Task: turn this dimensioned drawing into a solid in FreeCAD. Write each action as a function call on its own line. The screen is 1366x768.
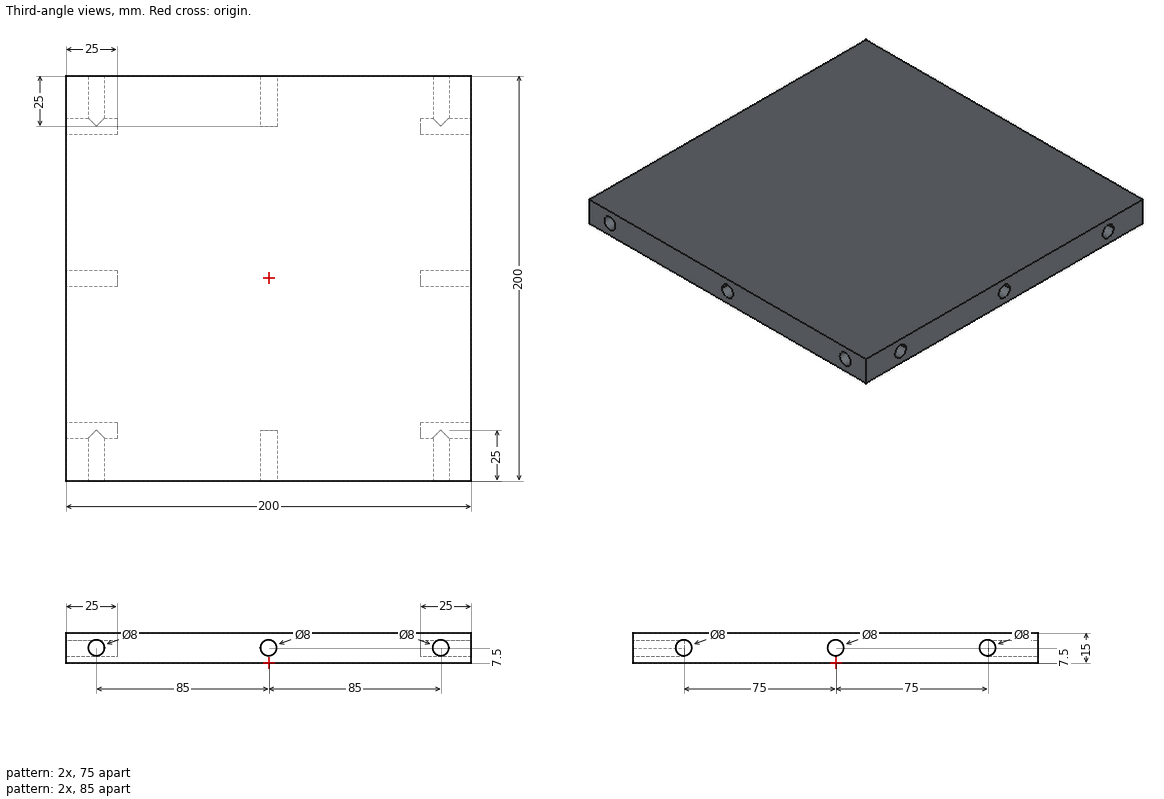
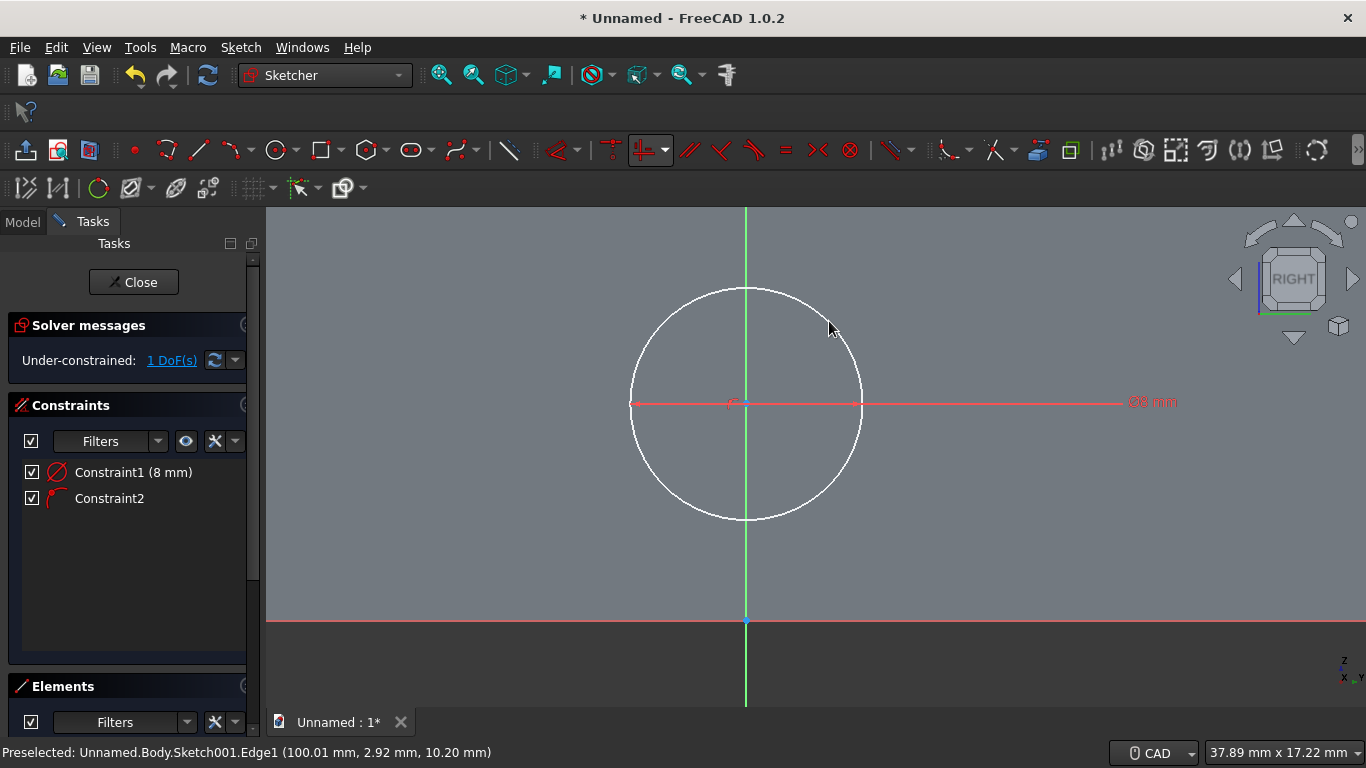
click(556, 150)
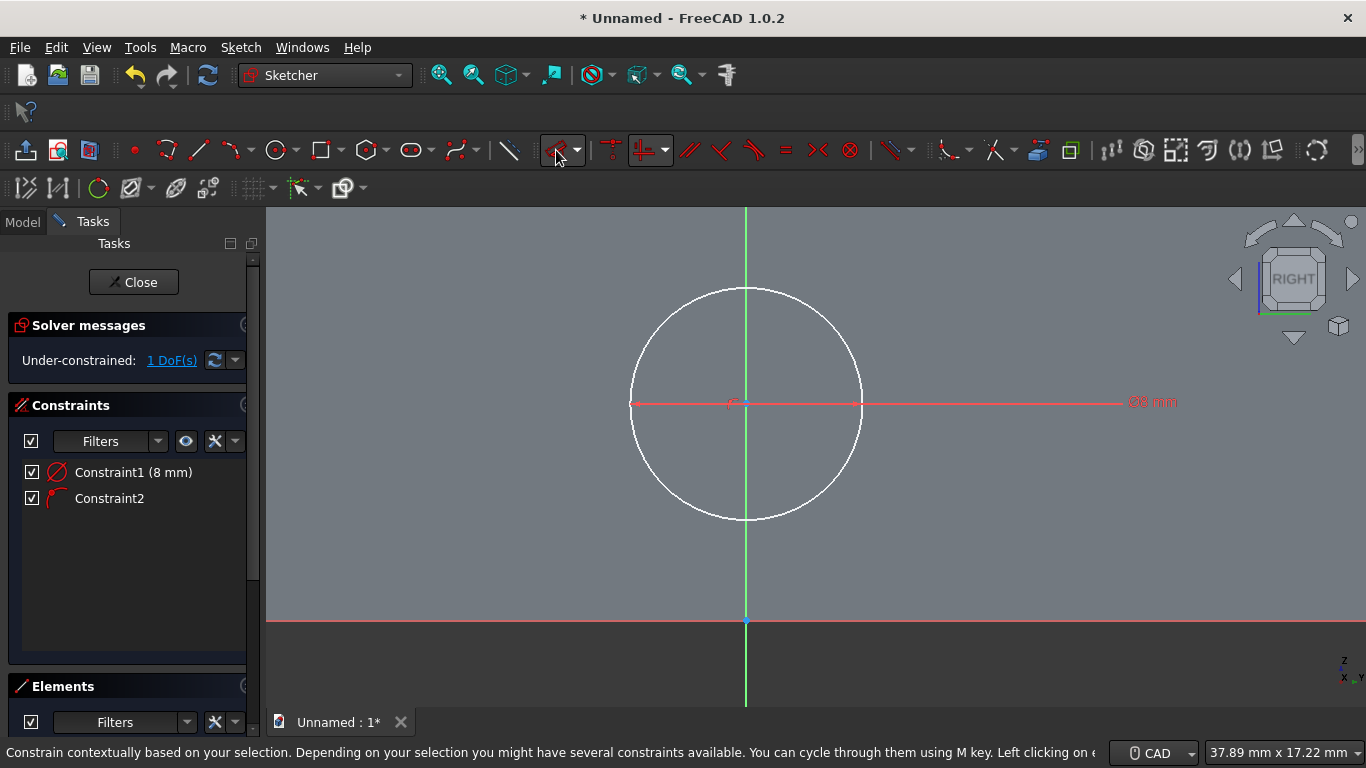
click(746, 404)
click(780, 462)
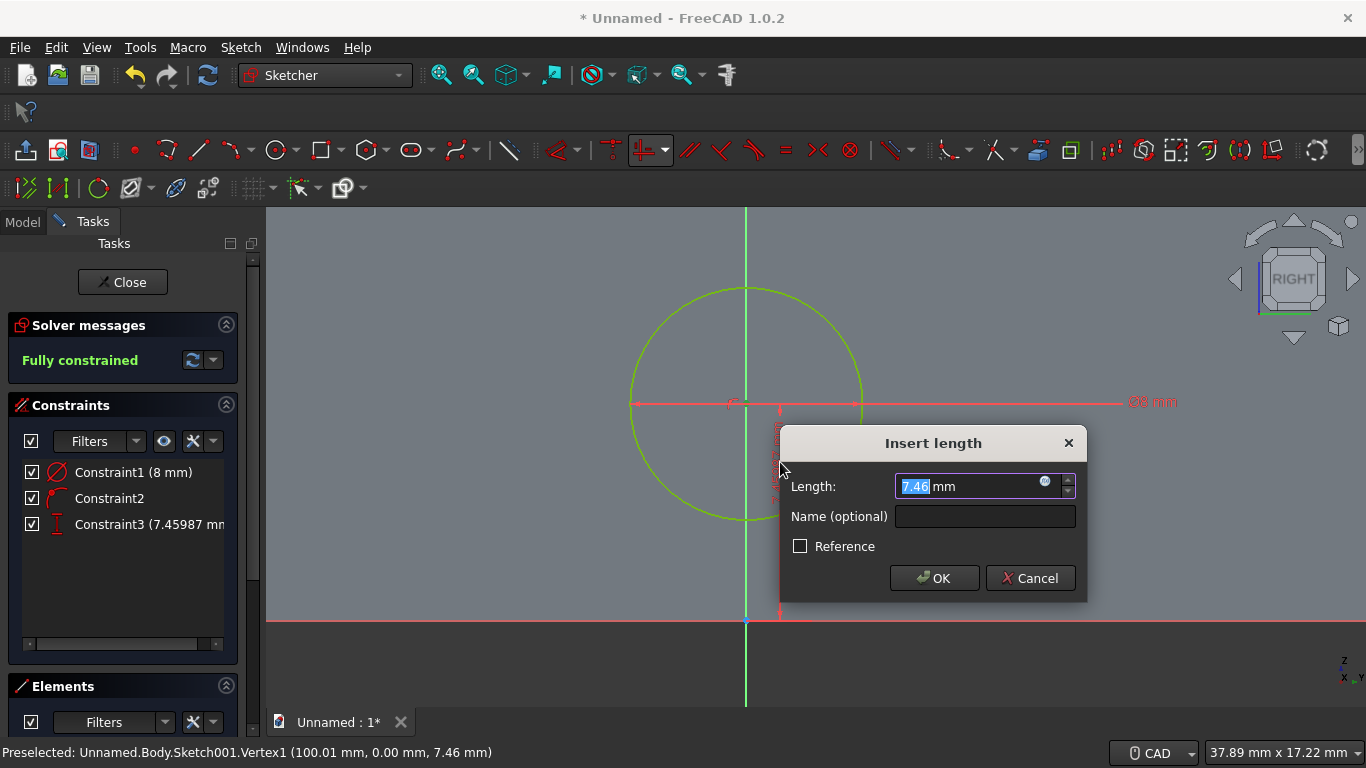
text(7.5)
key(Return)
key(Escape)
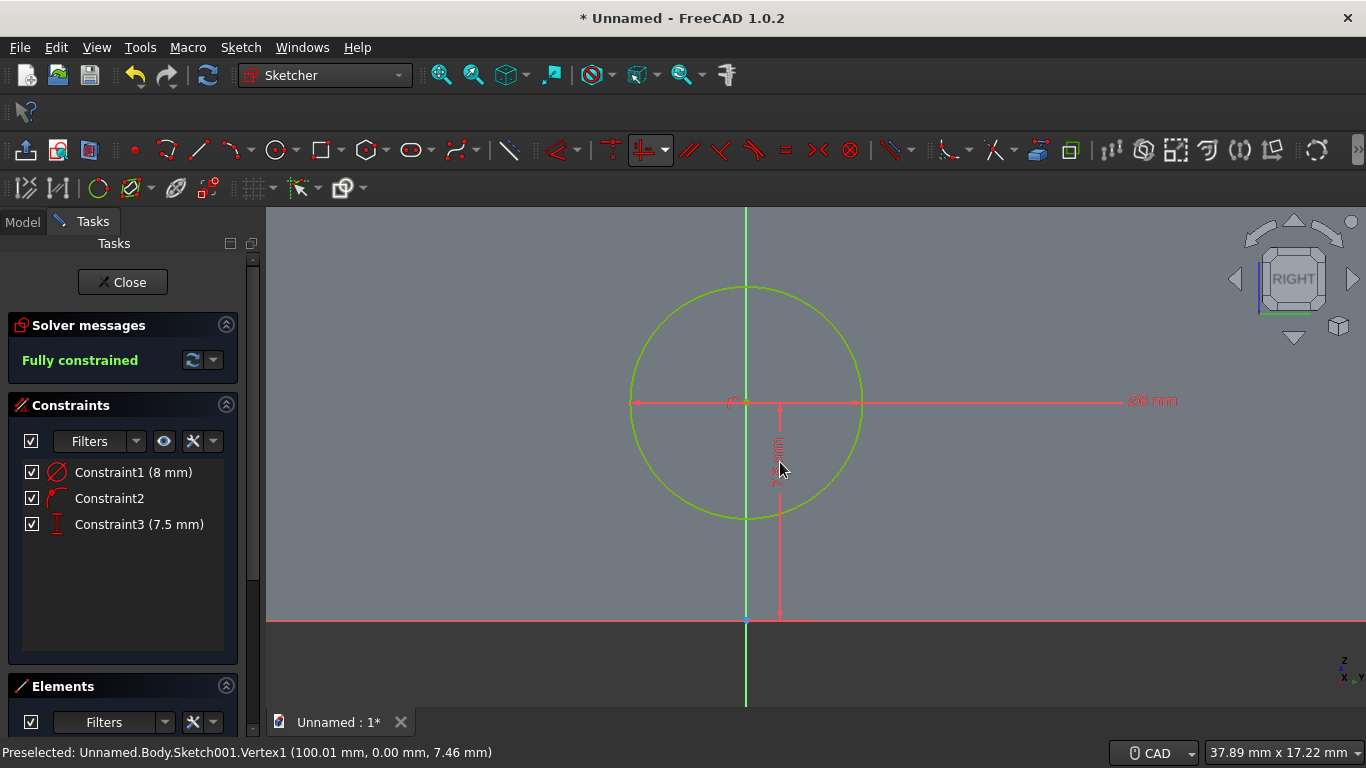
click(123, 282)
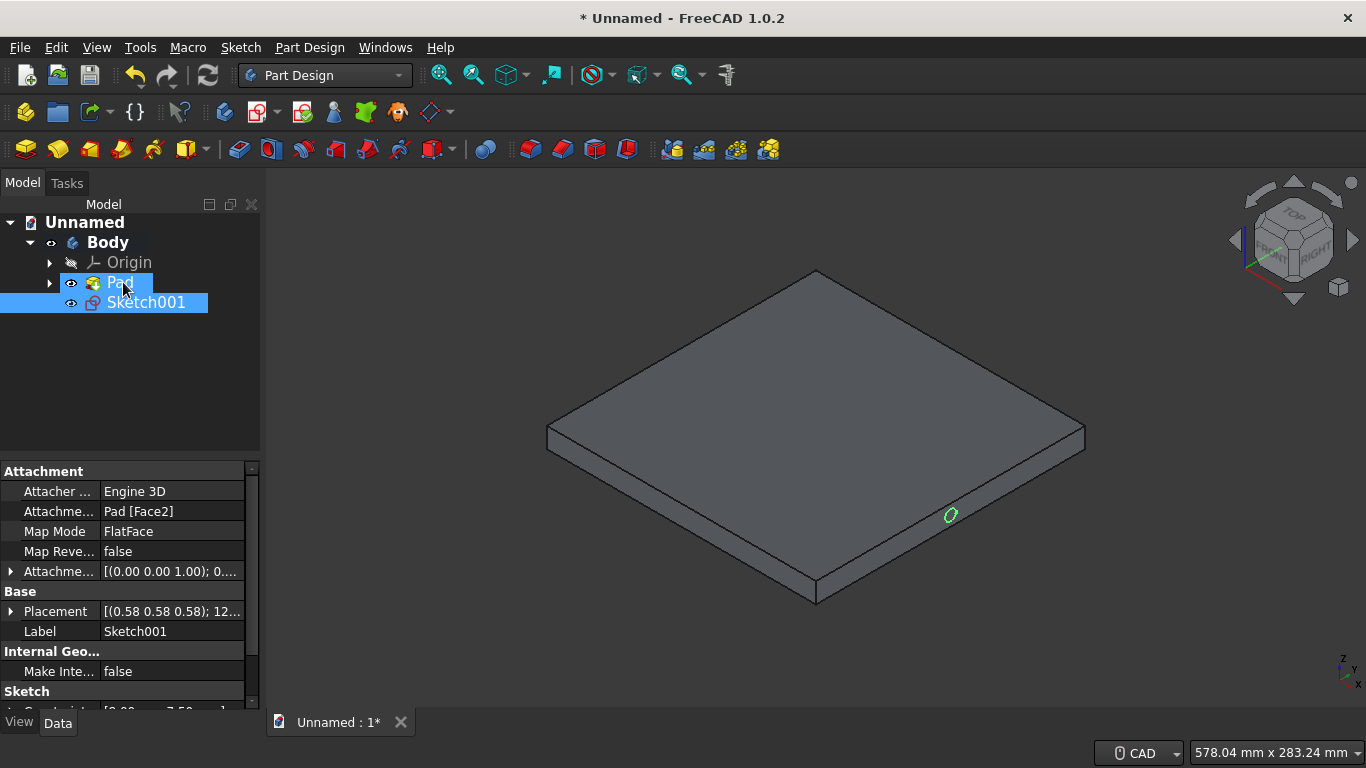
click(240, 150)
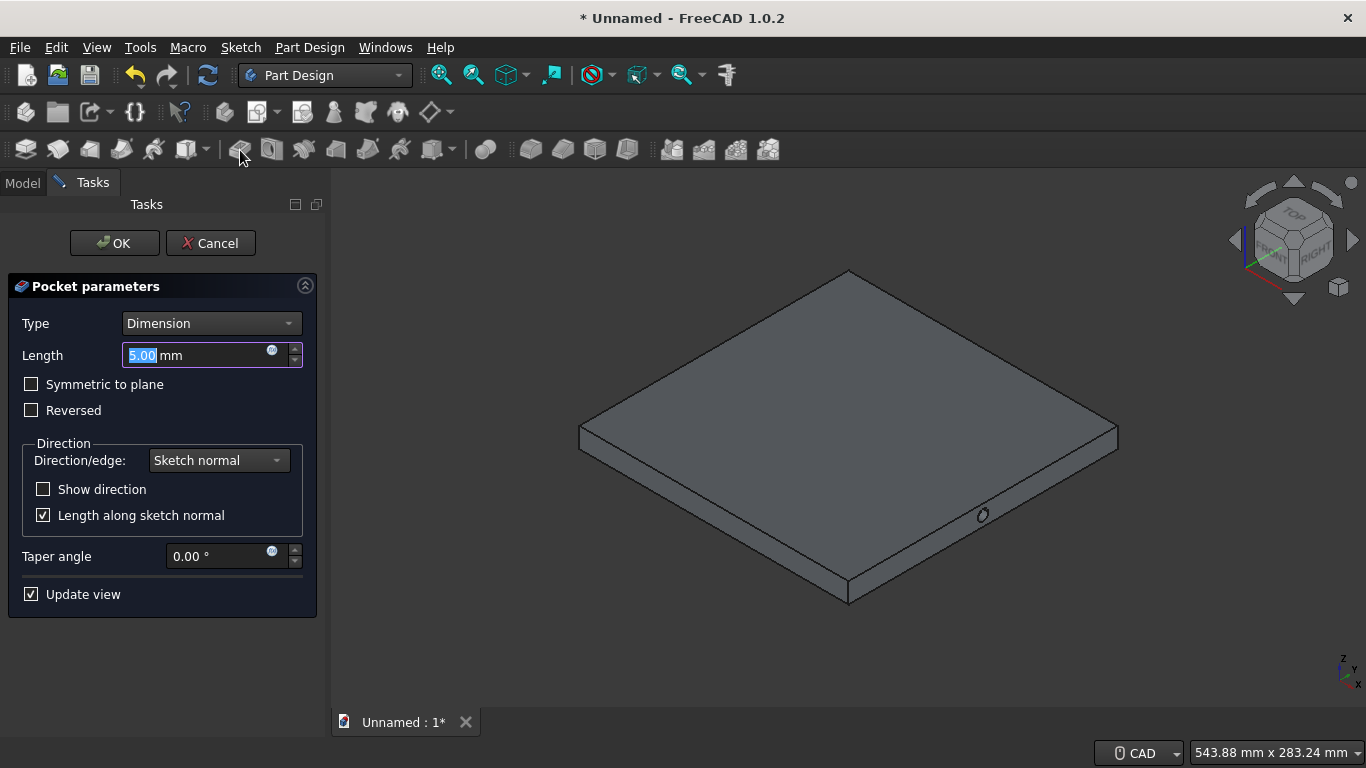
text(25)
key(Tab)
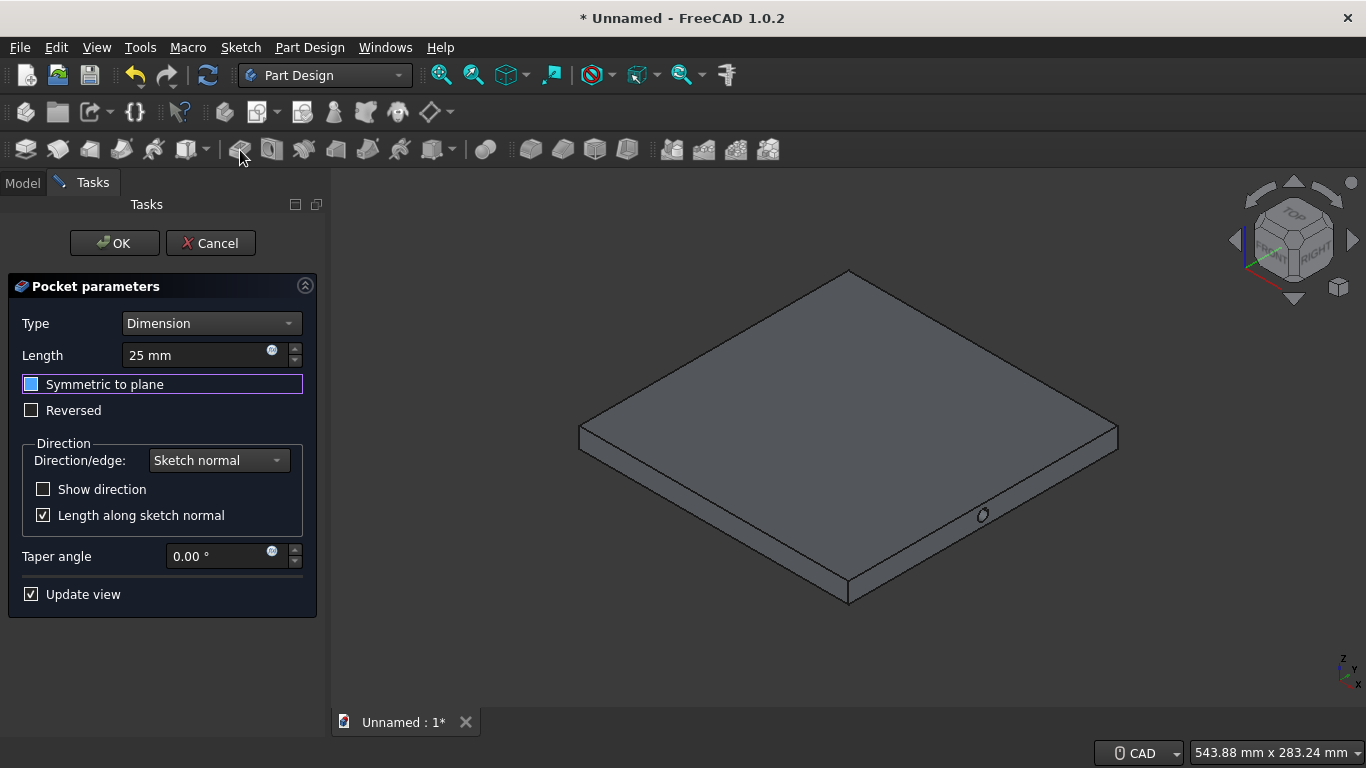
click(115, 243)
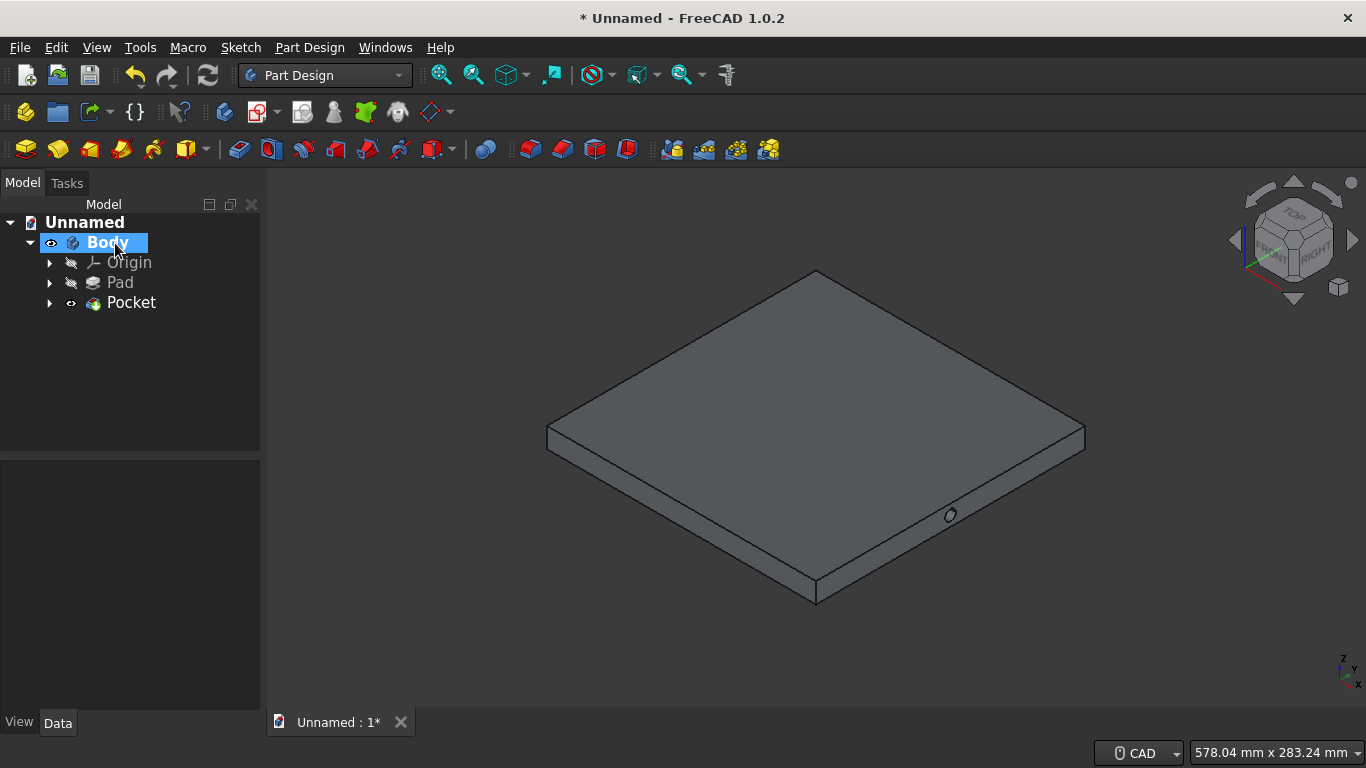
click(116, 303)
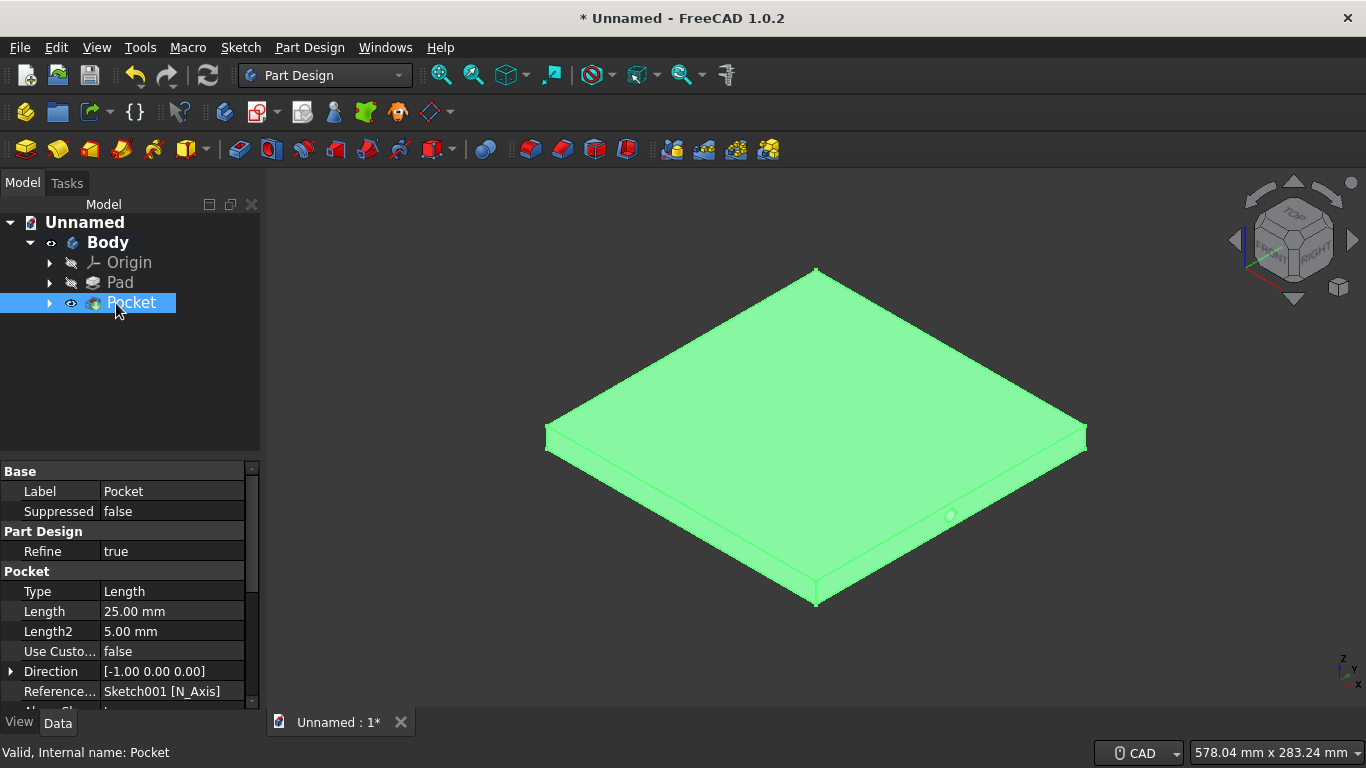
click(704, 150)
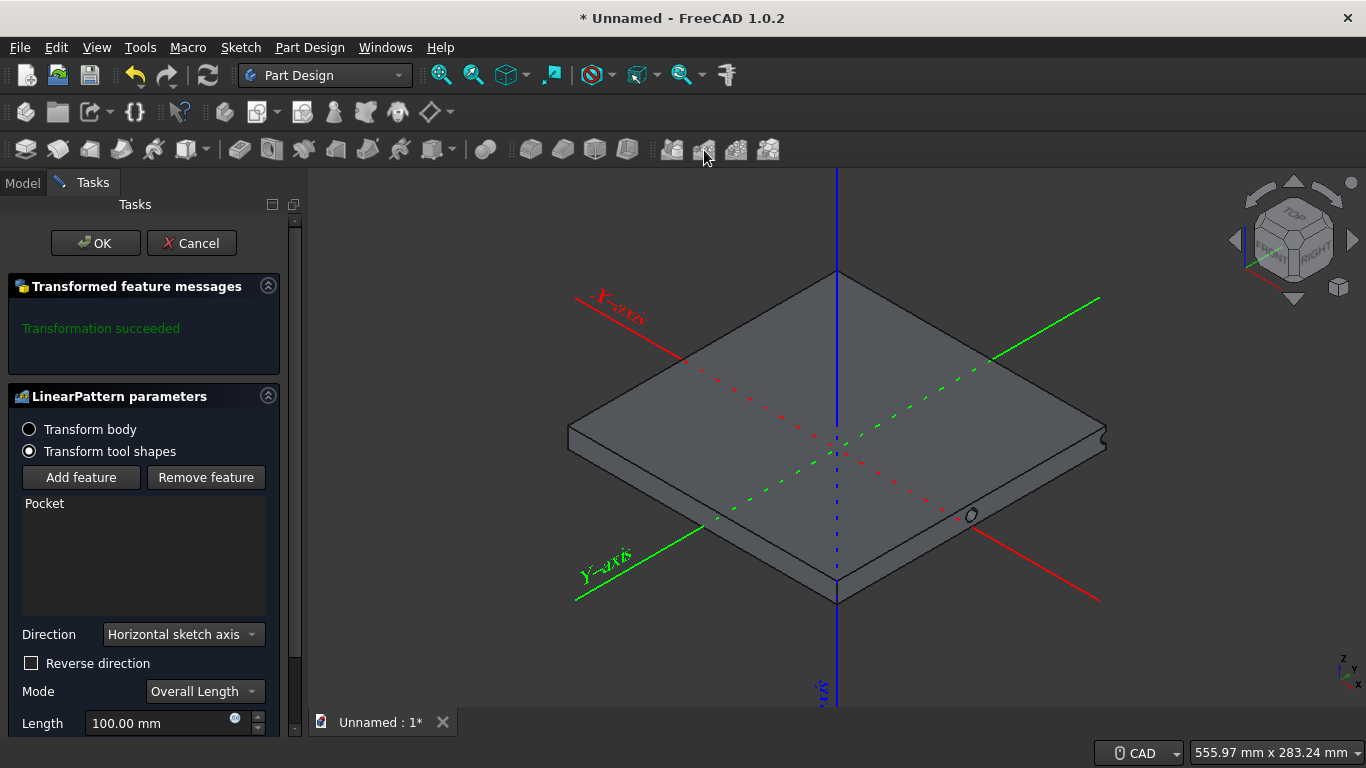
click(184, 634)